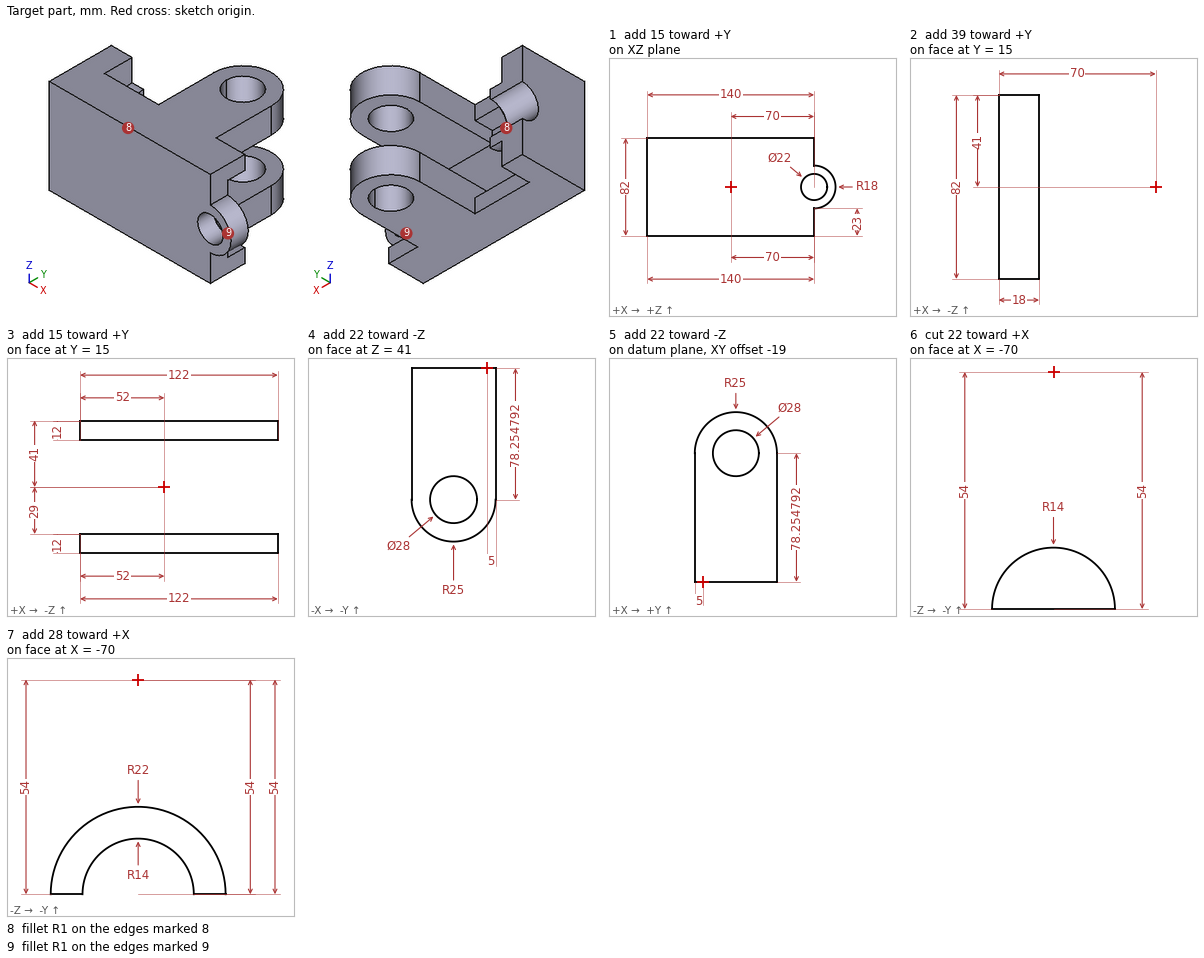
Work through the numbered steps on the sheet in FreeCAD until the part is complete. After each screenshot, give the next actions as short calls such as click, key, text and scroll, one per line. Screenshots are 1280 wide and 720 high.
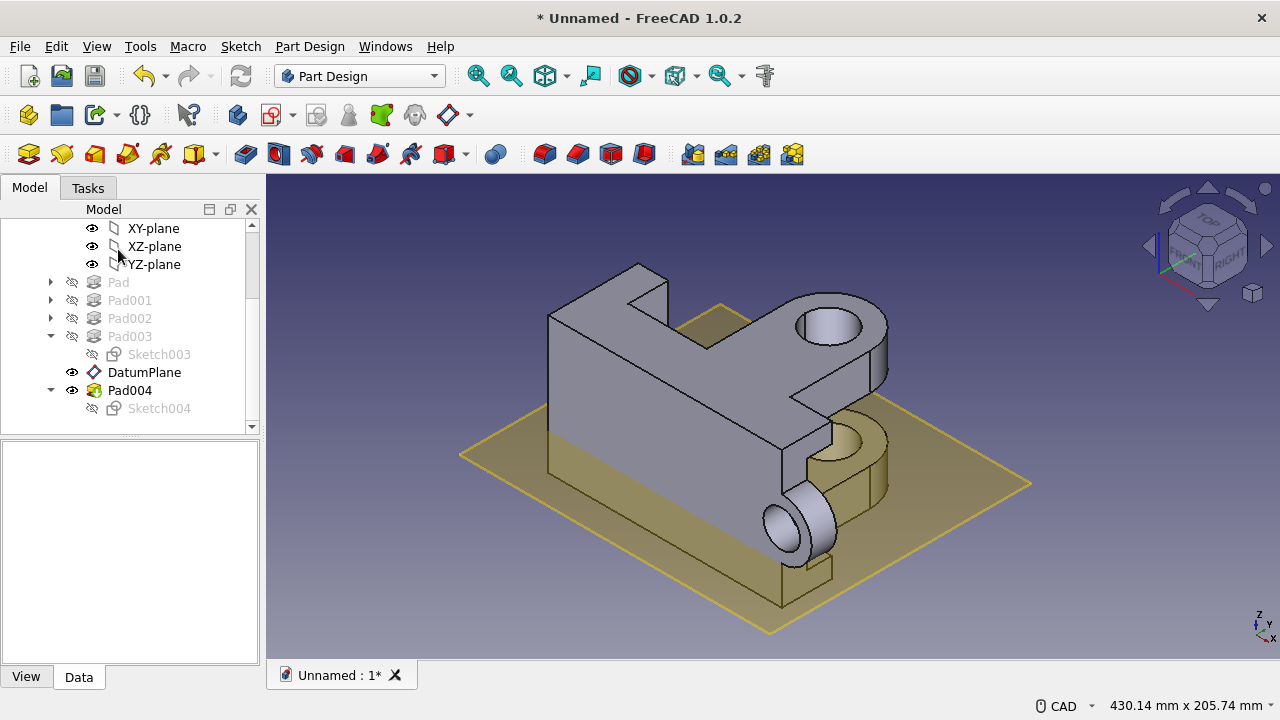
click(117, 372)
key(space)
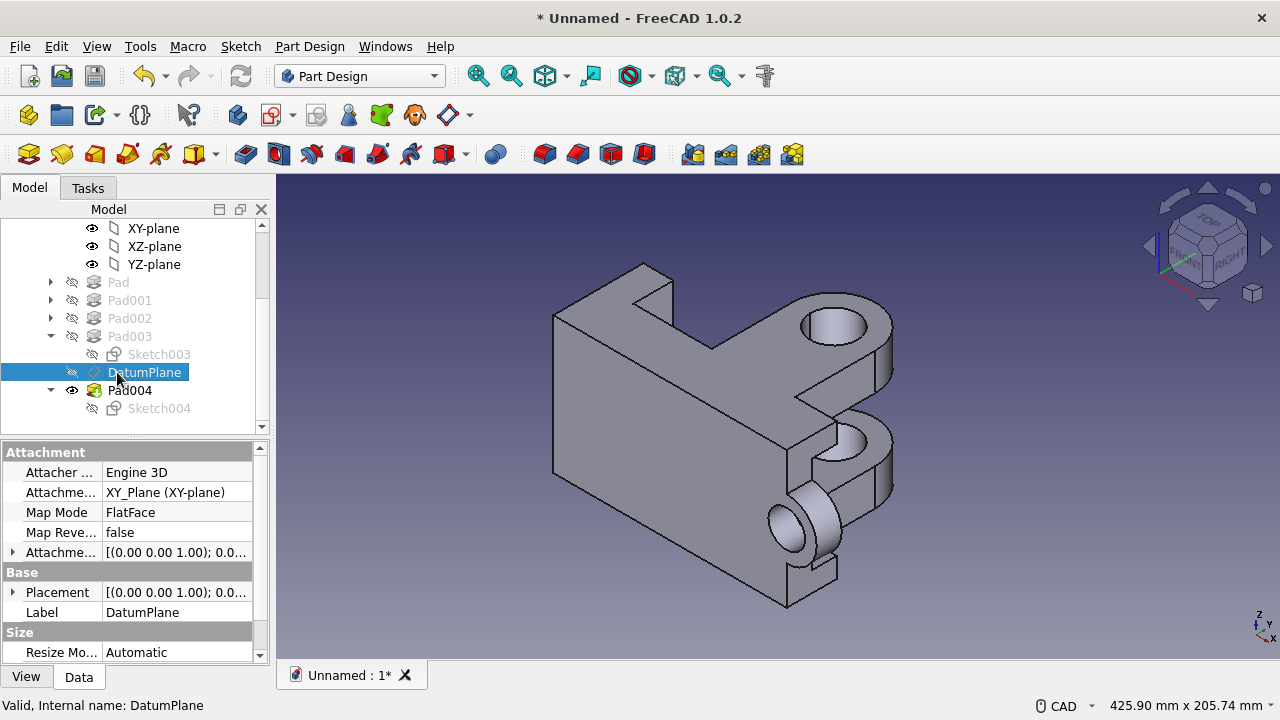
key(6)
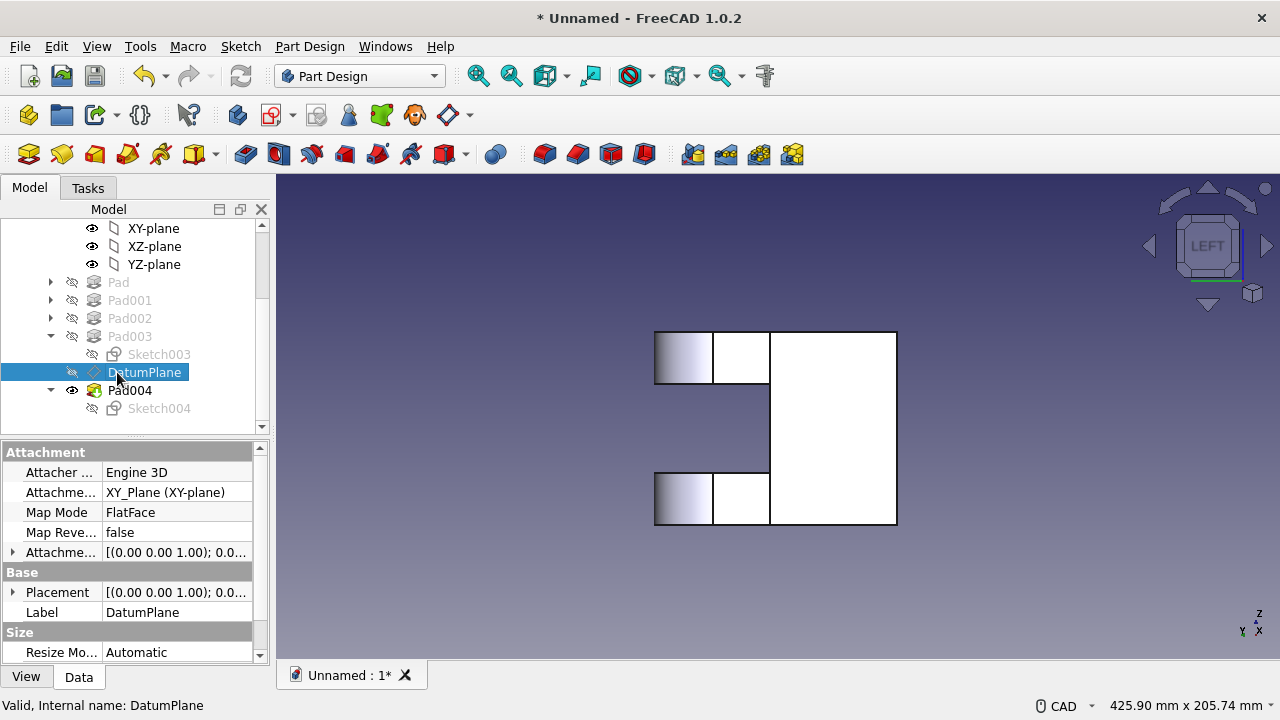
click(479, 76)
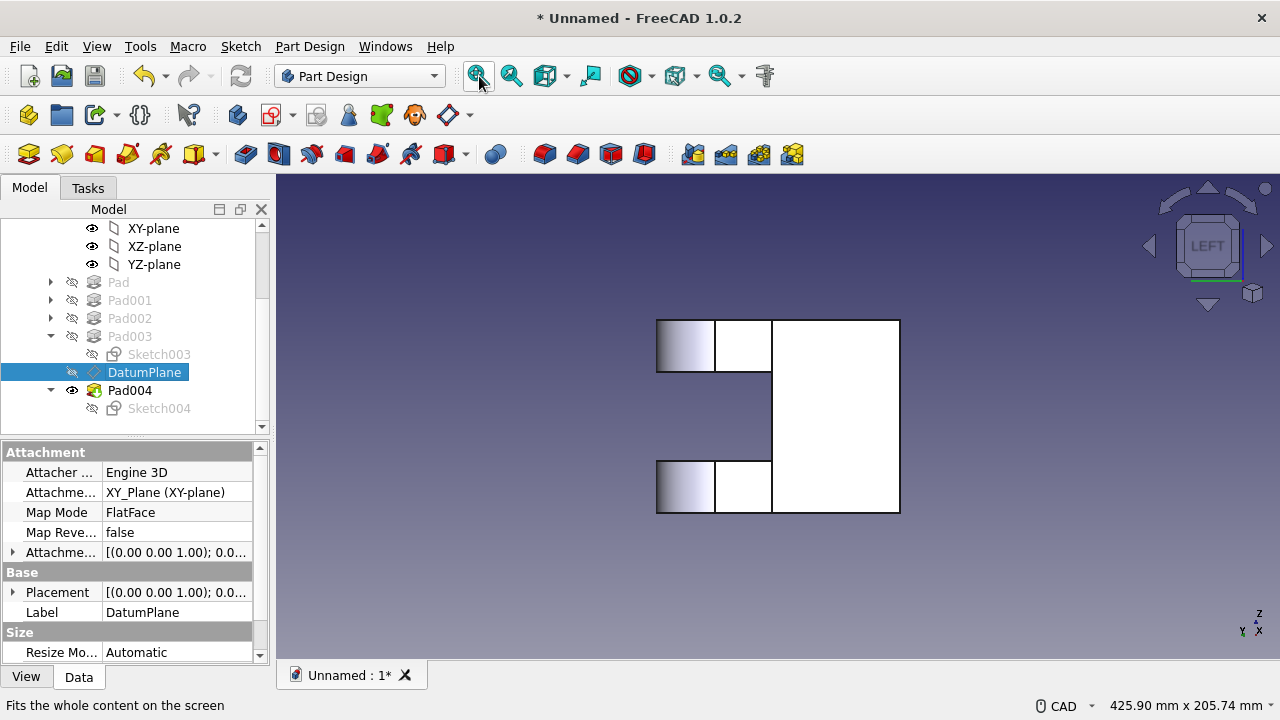
click(836, 443)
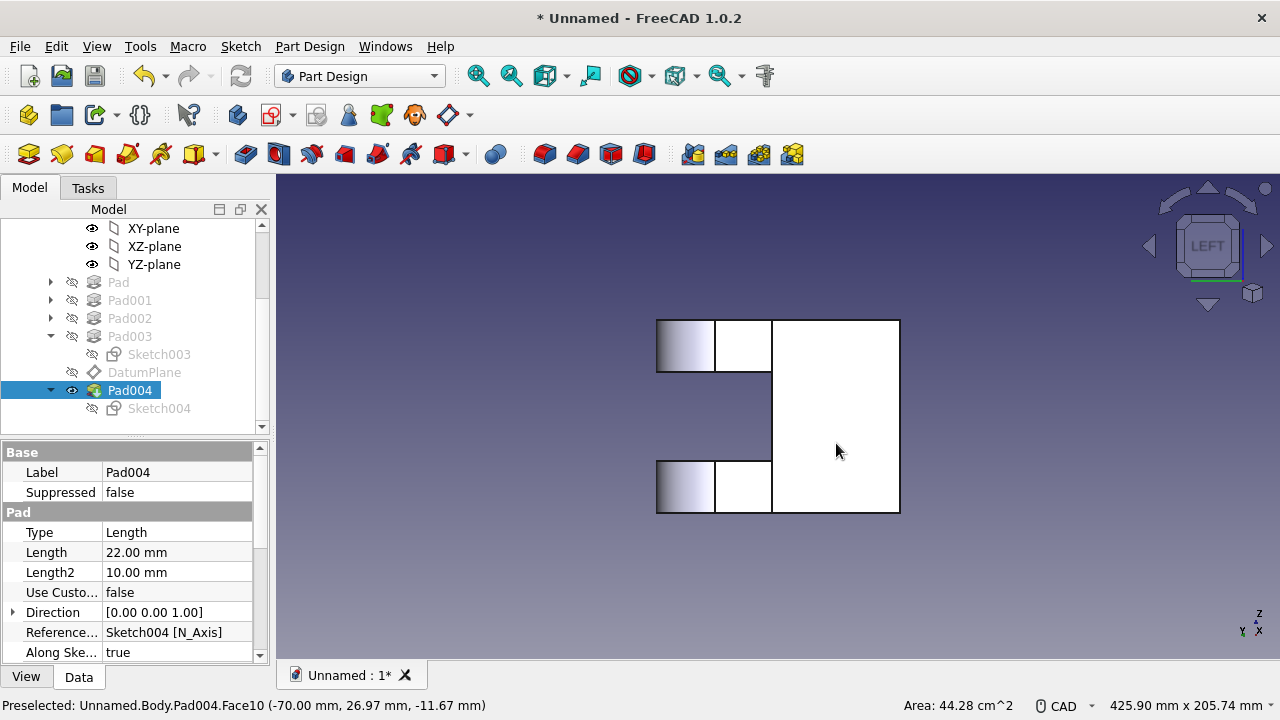
click(270, 116)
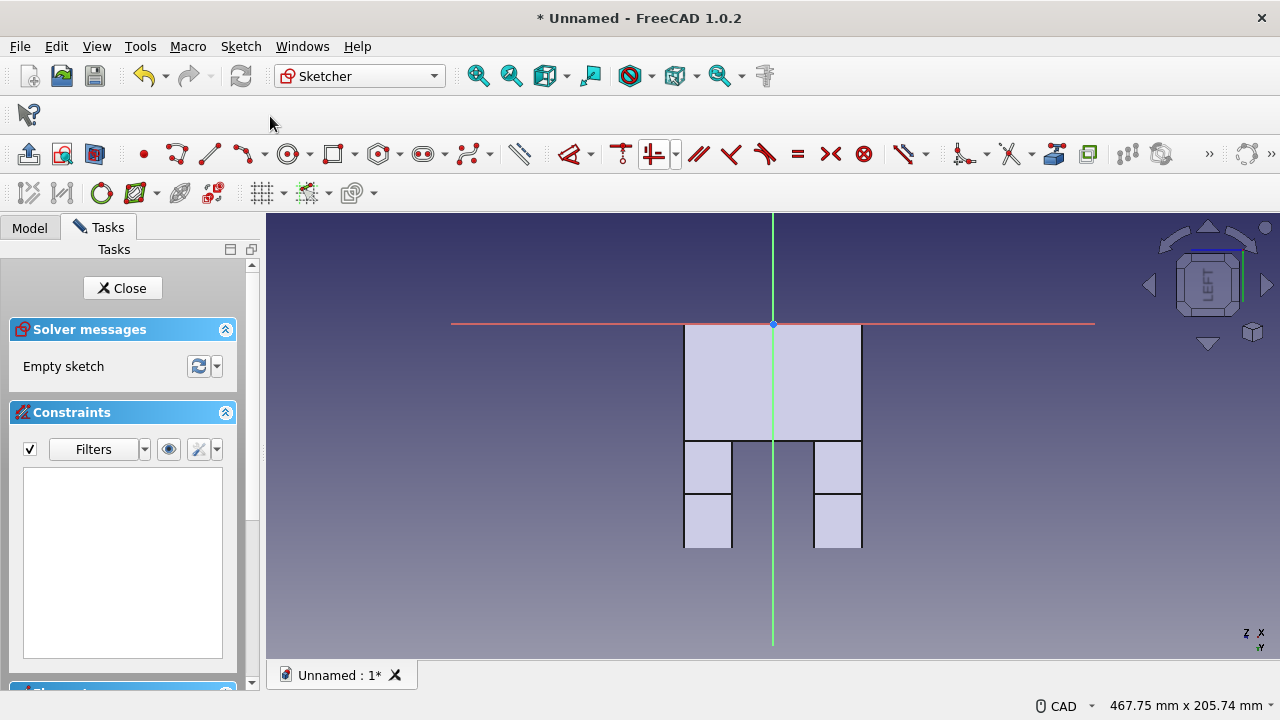
scroll(829, 339, up, 4)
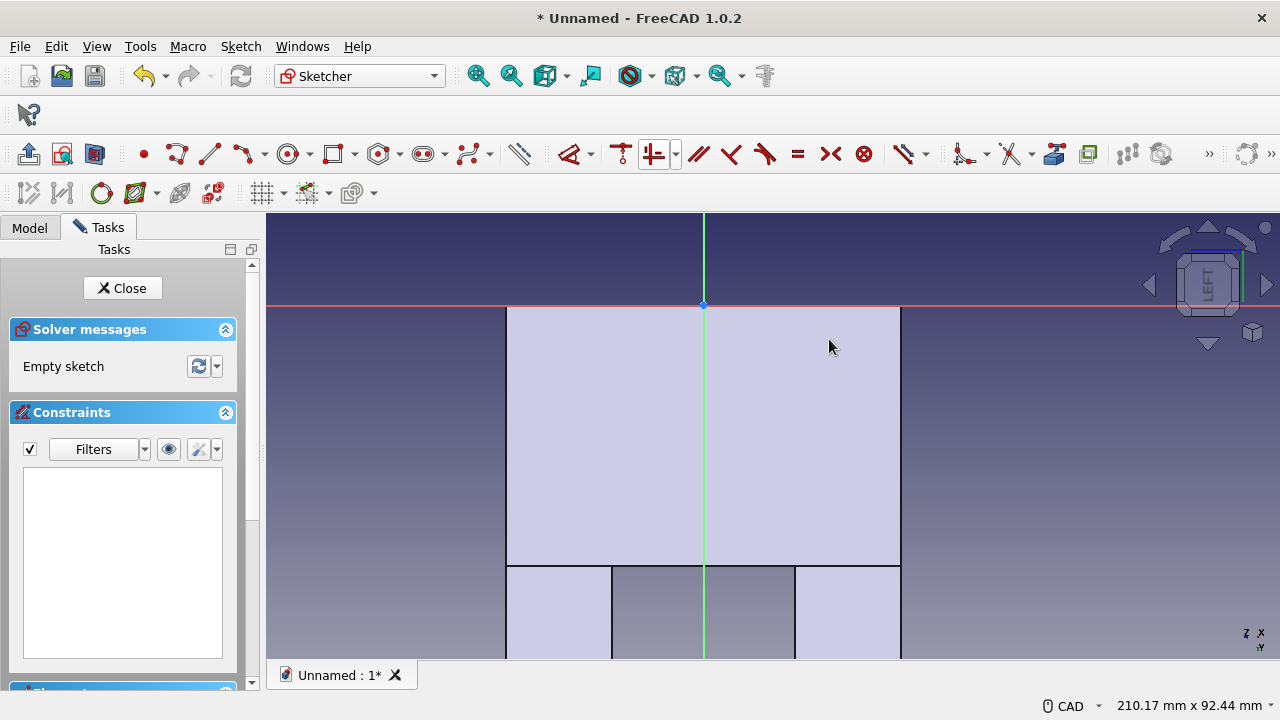
click(210, 154)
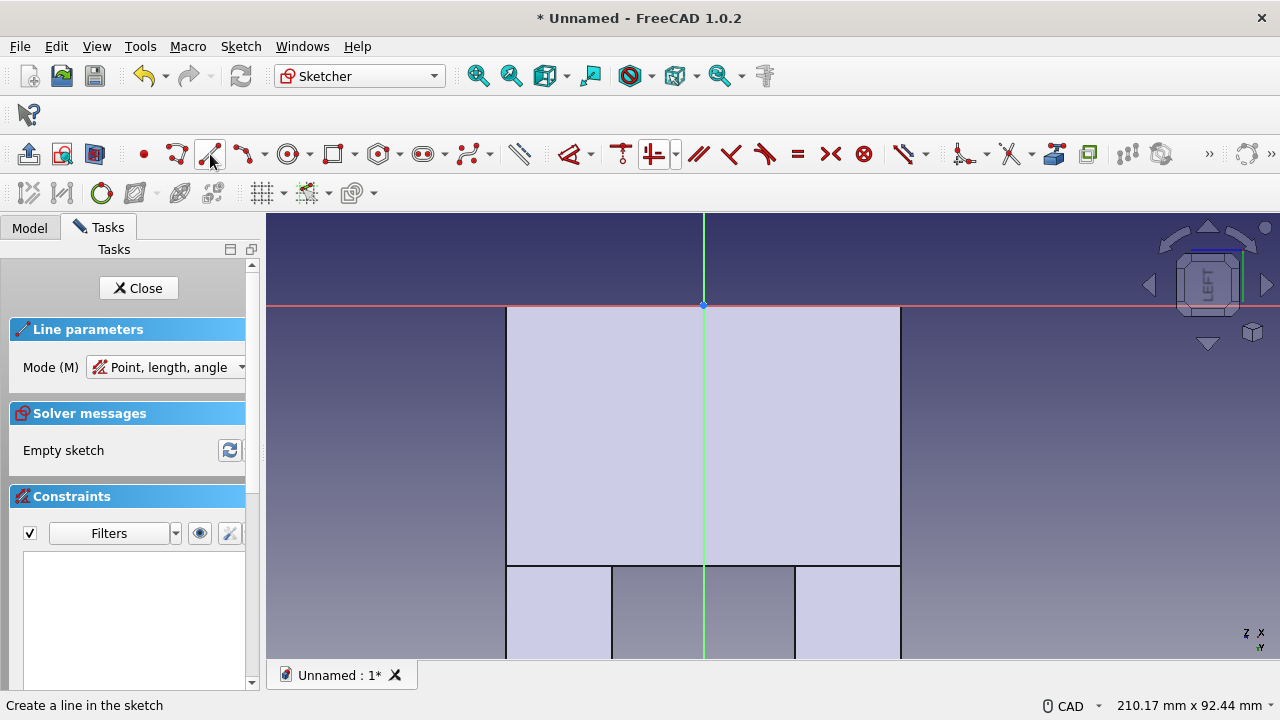
click(636, 566)
click(771, 566)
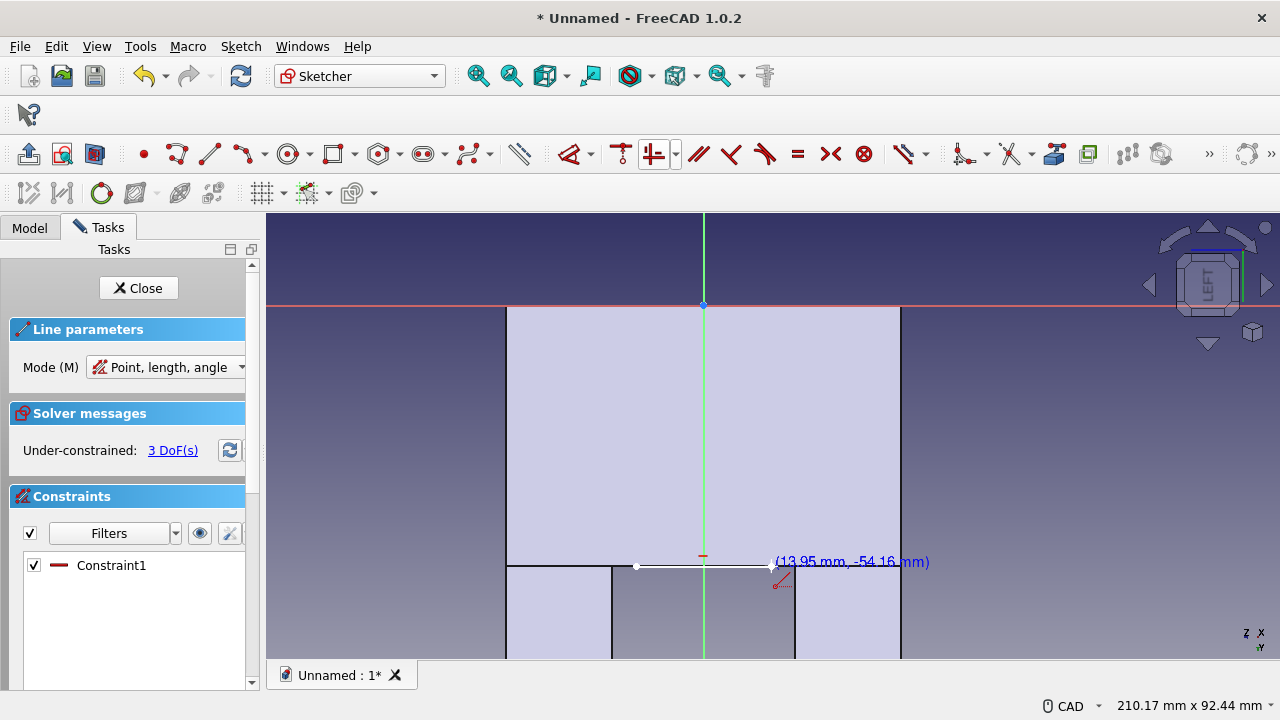
click(242, 154)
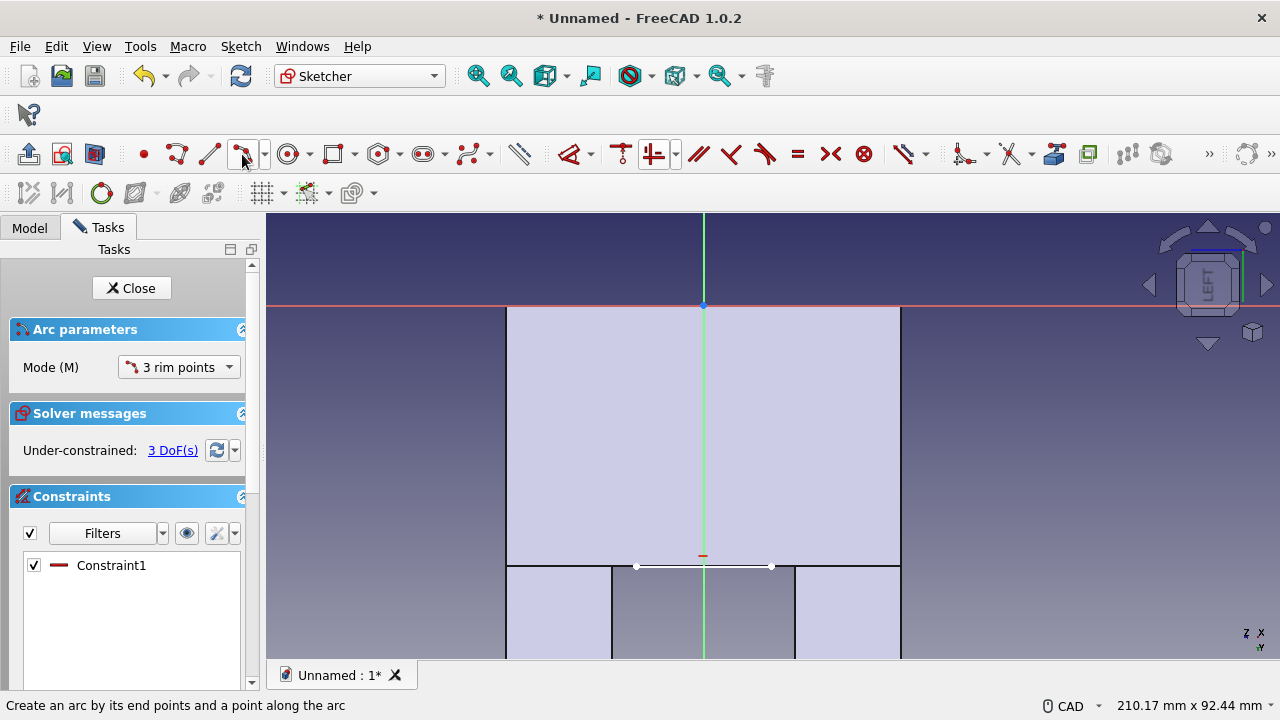
click(771, 567)
click(636, 567)
click(725, 502)
key(Escape)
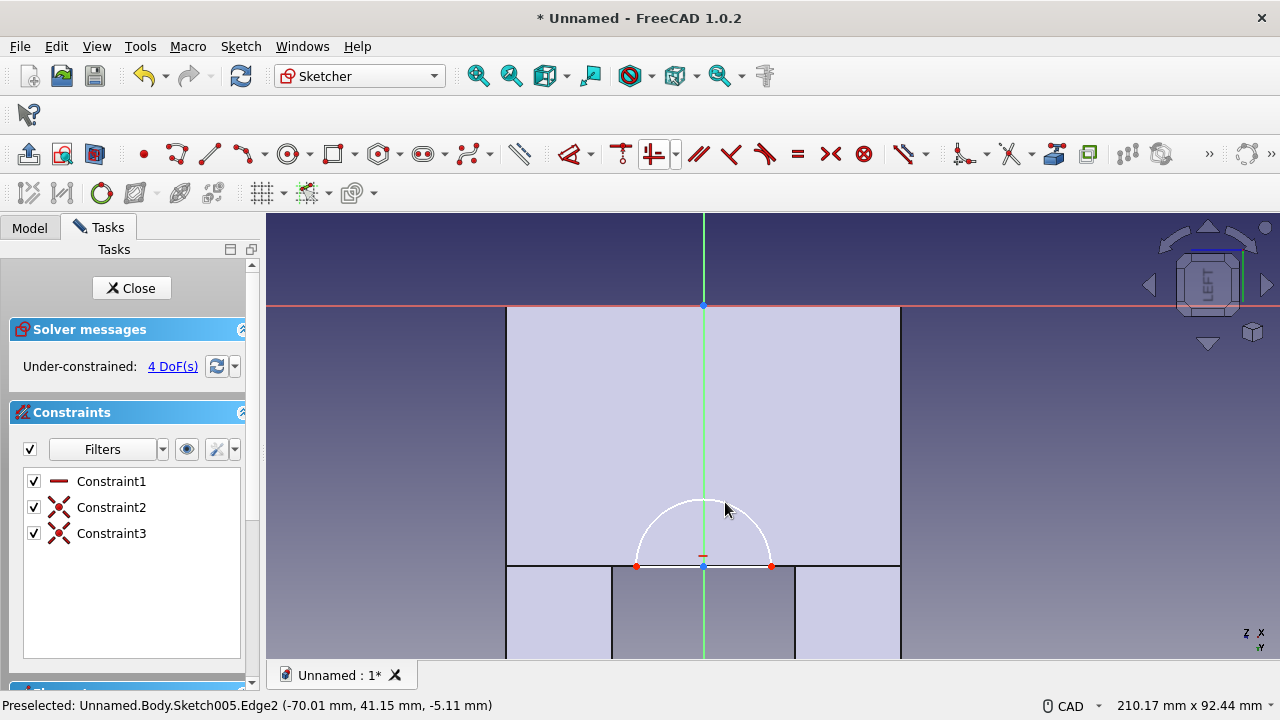
click(704, 567)